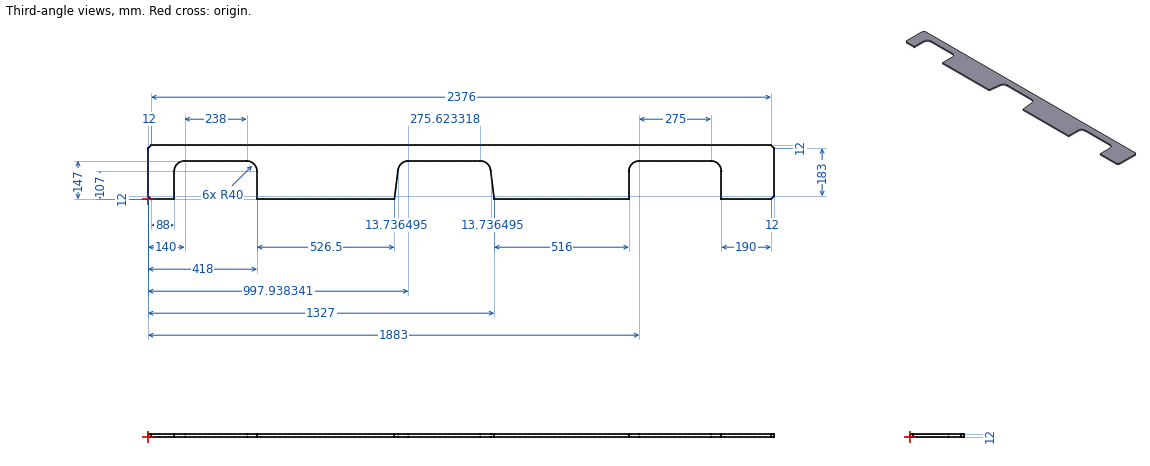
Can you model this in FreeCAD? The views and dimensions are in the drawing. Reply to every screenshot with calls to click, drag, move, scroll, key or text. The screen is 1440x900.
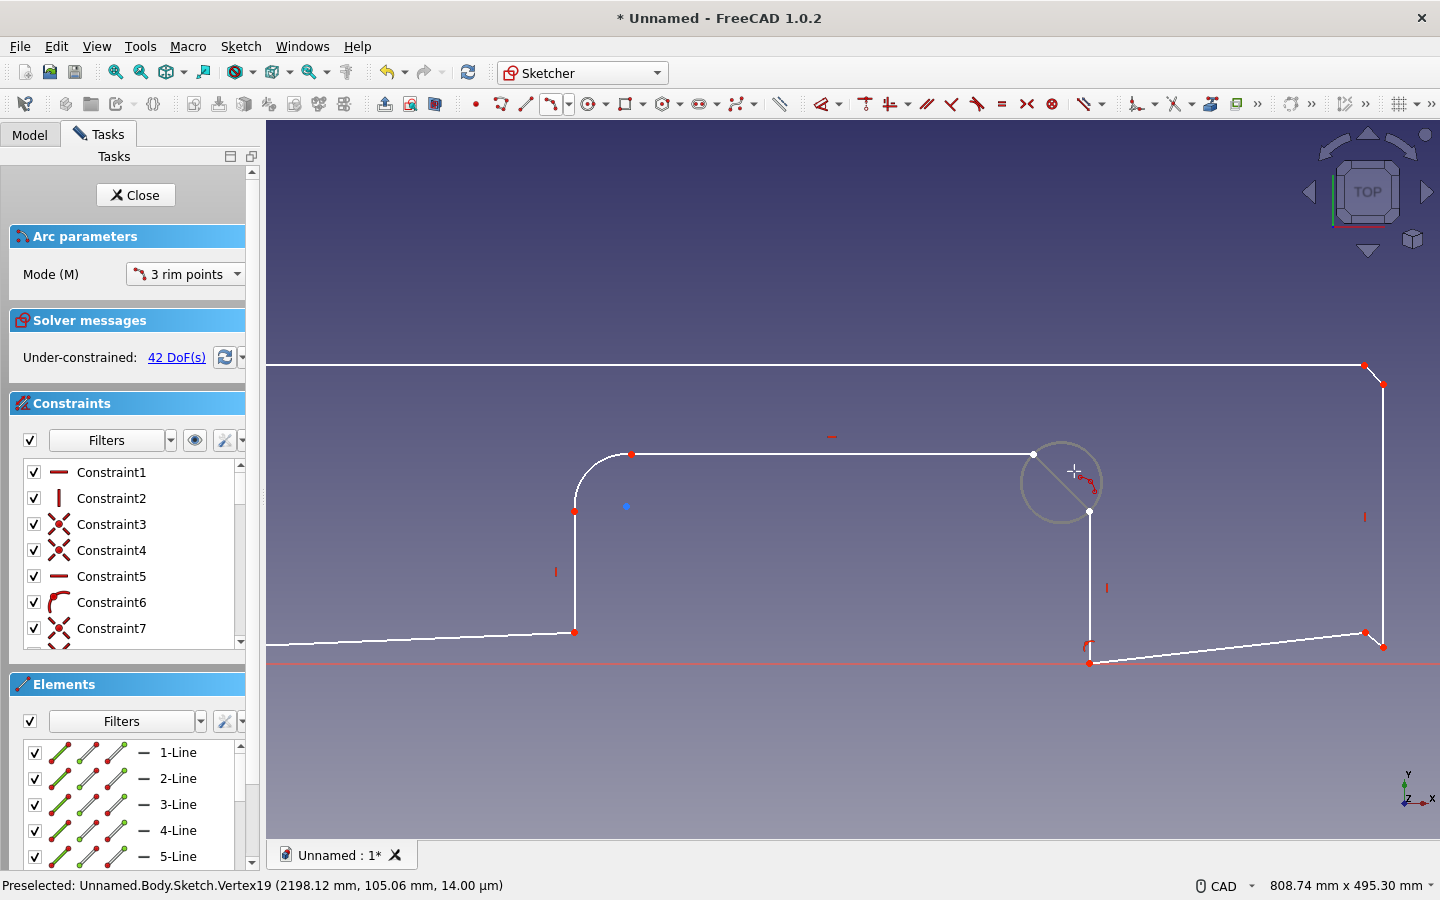
click(1073, 467)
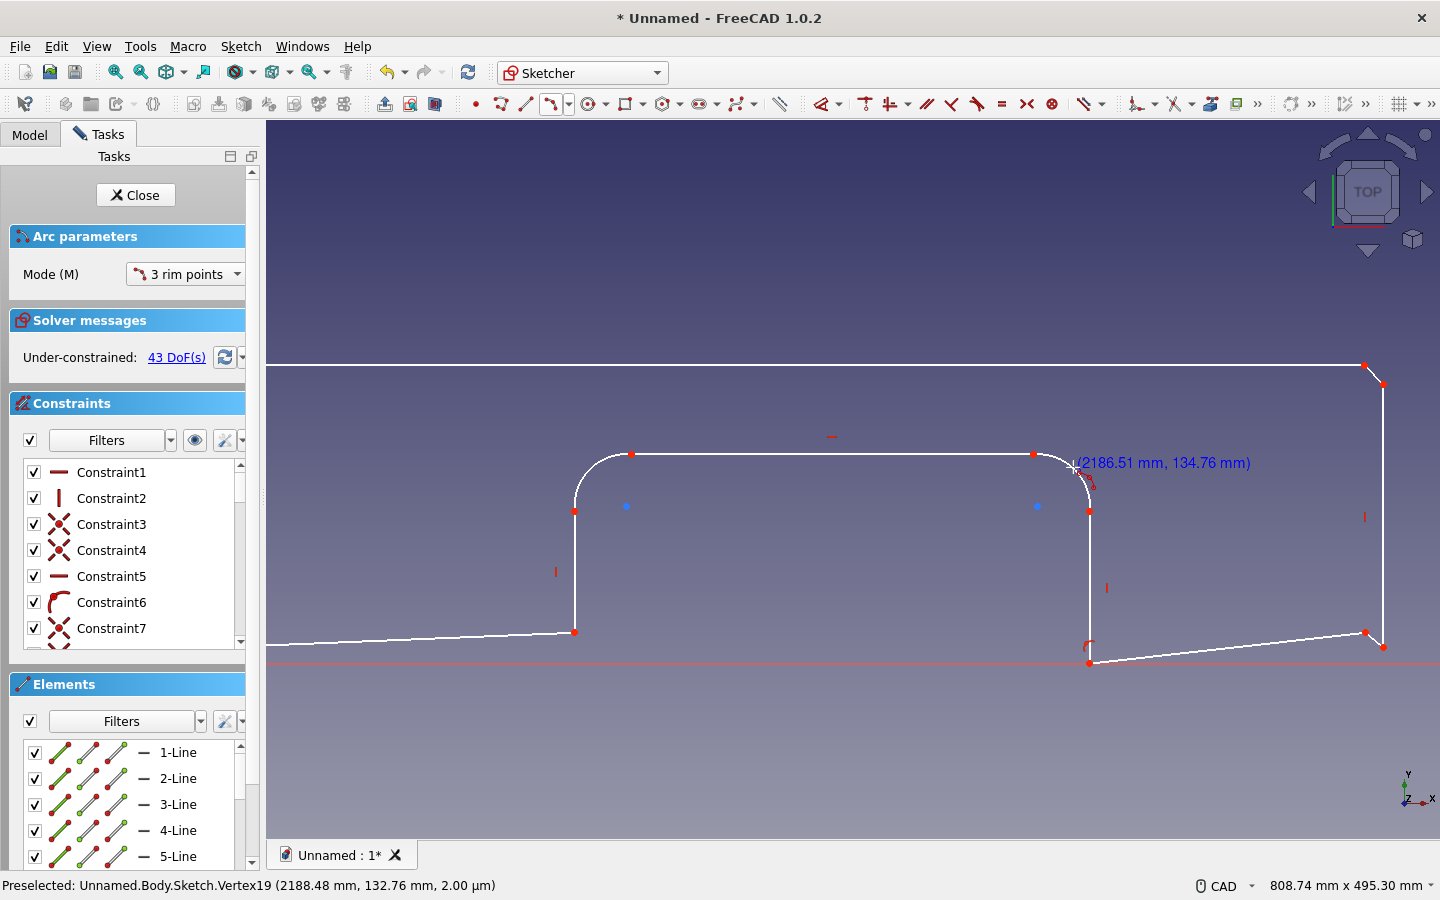
scroll(1074, 471, down, 8)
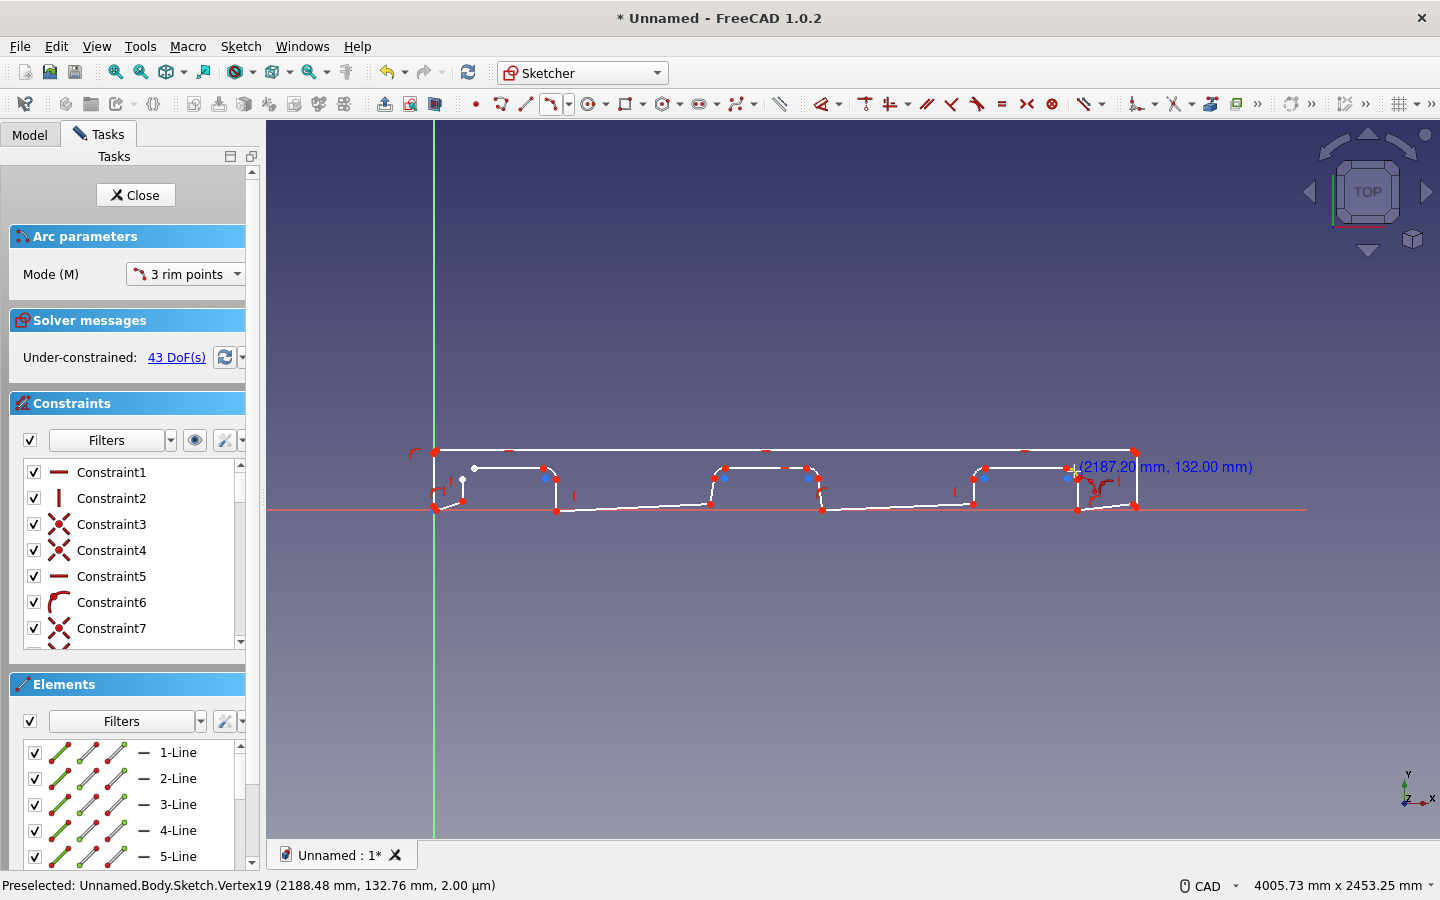
click(463, 480)
click(474, 468)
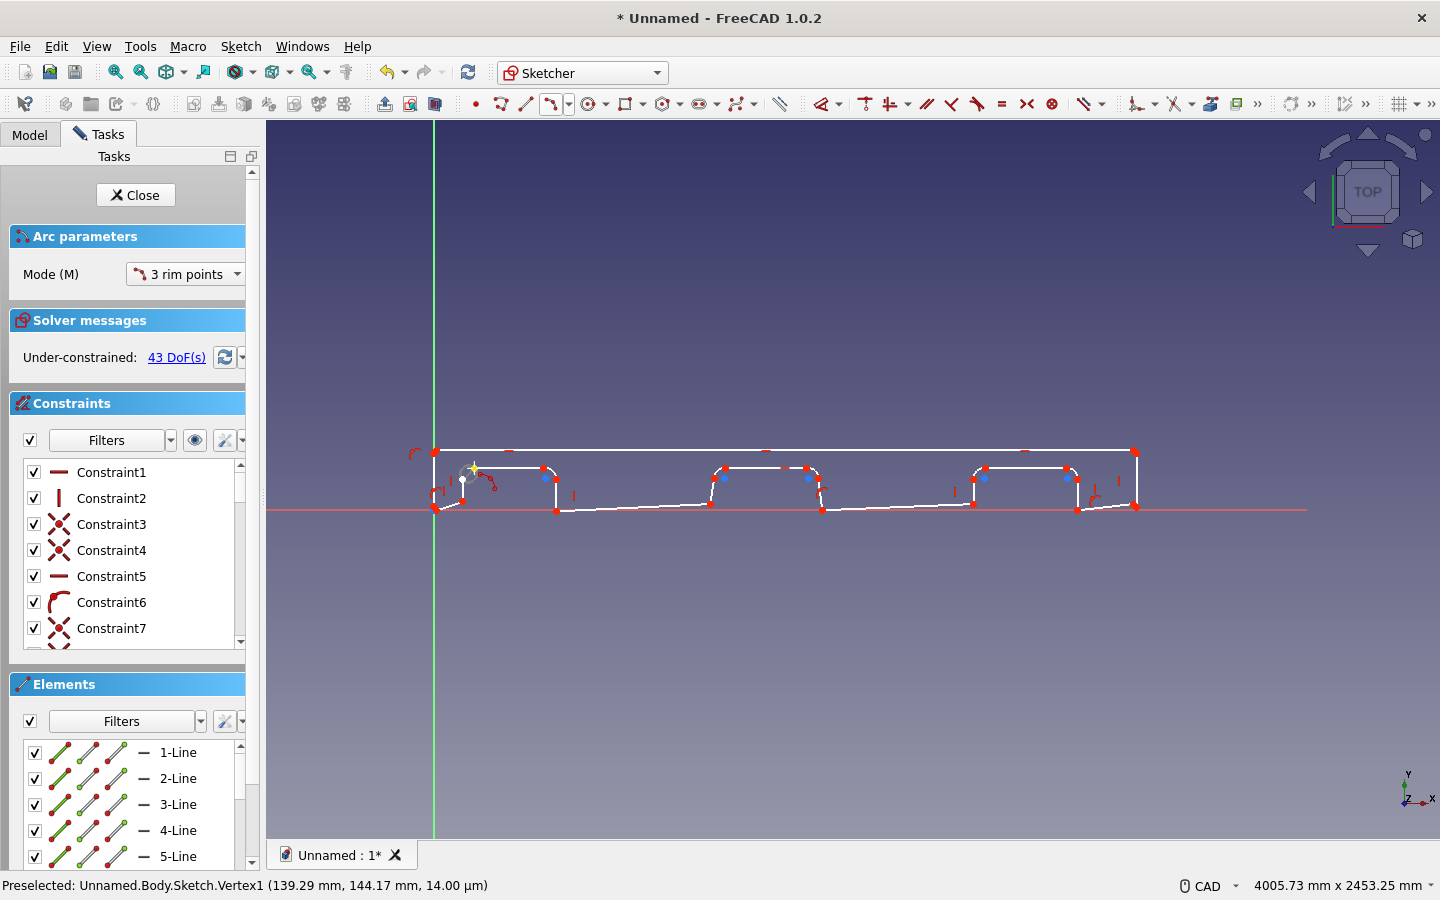
scroll(466, 471, up, 8)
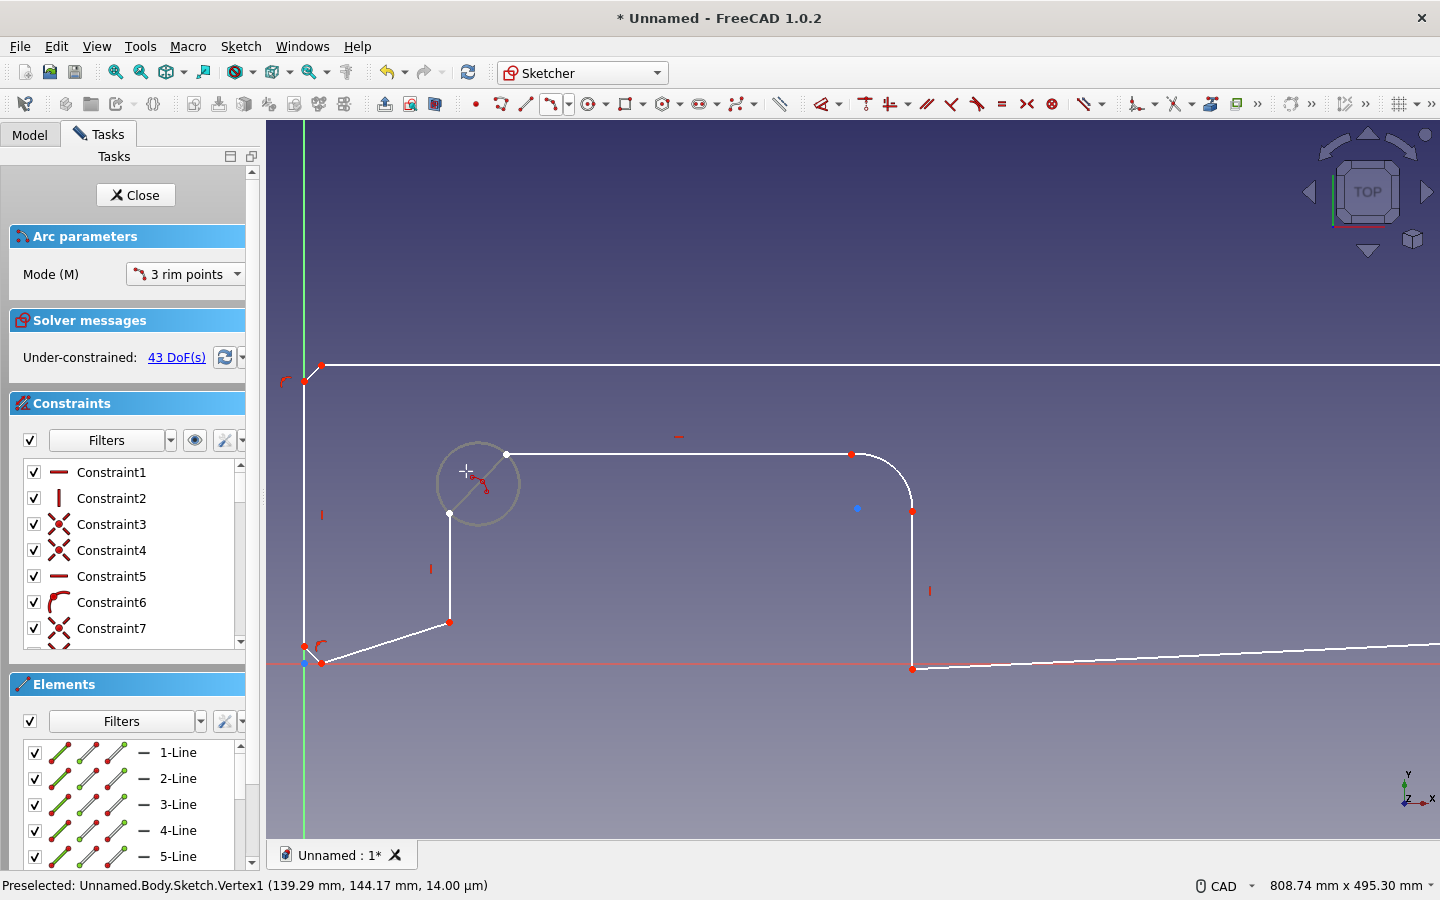
click(467, 467)
key(Escape)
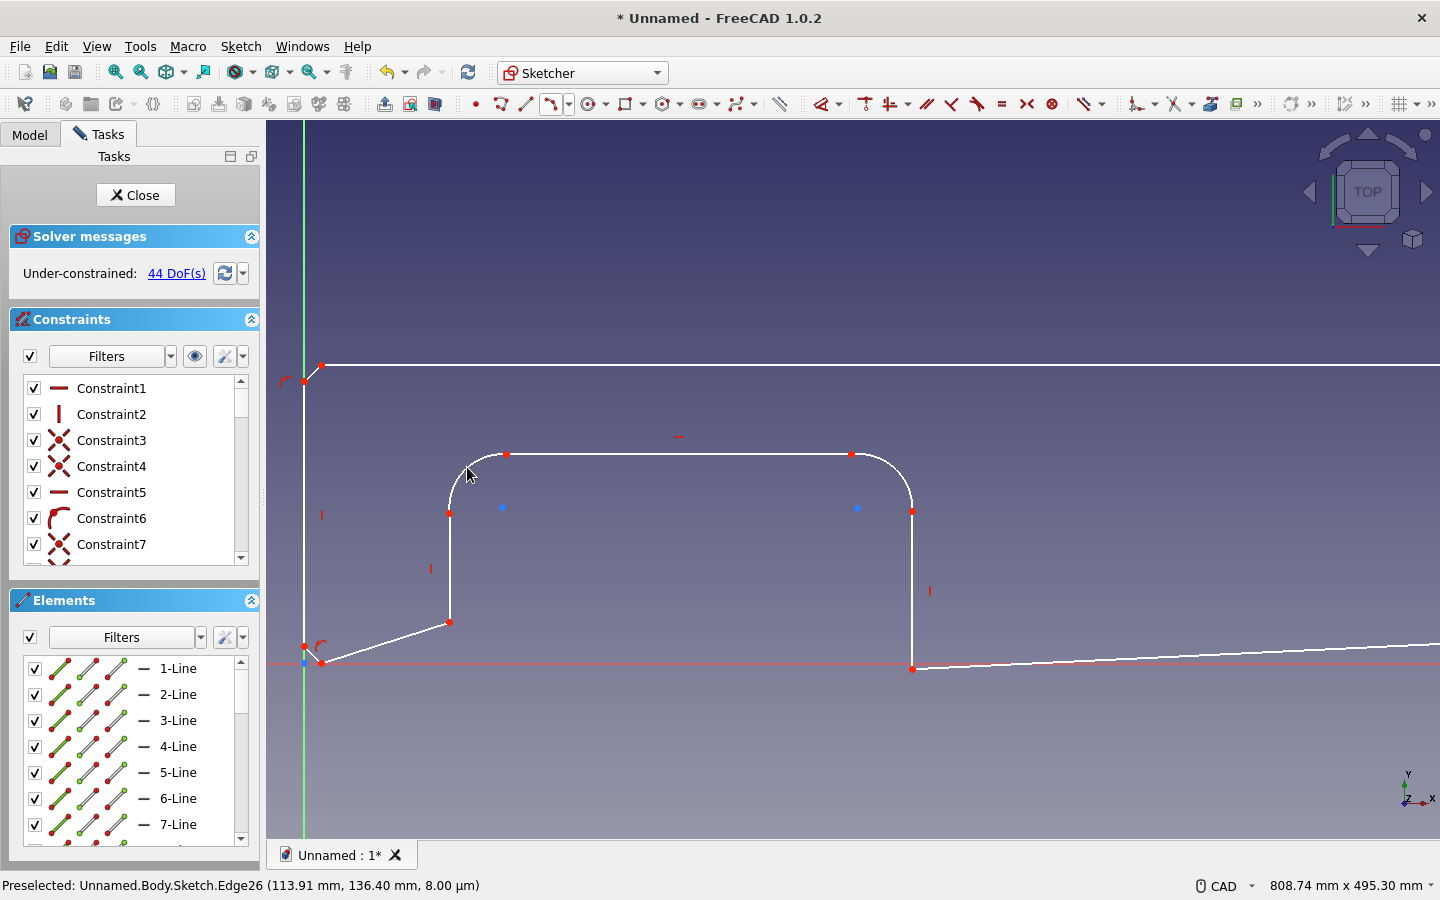
scroll(465, 471, down, 8)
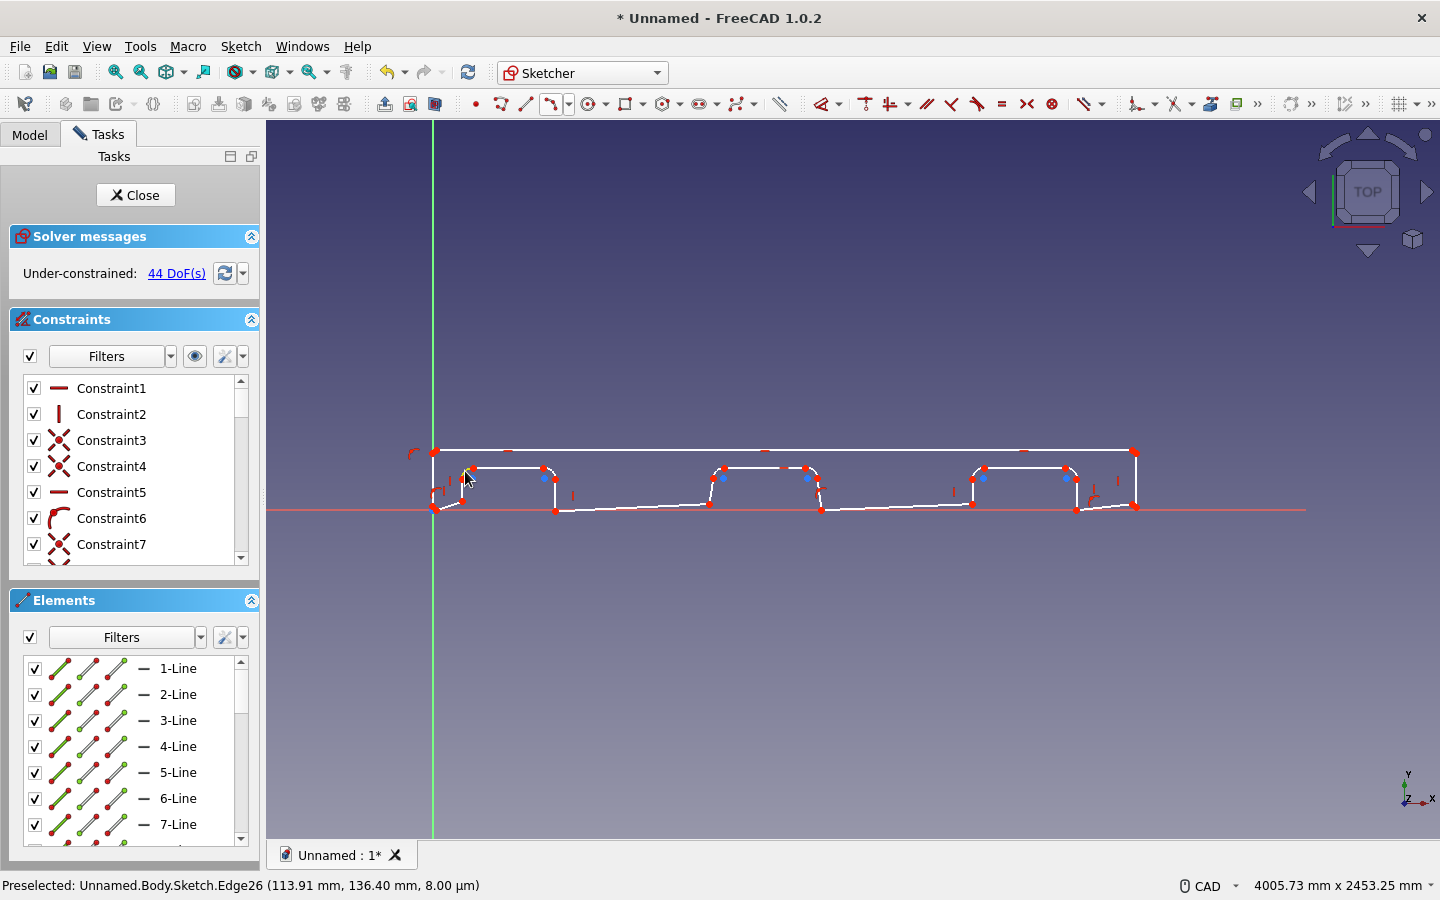
scroll(711, 496, up, 3)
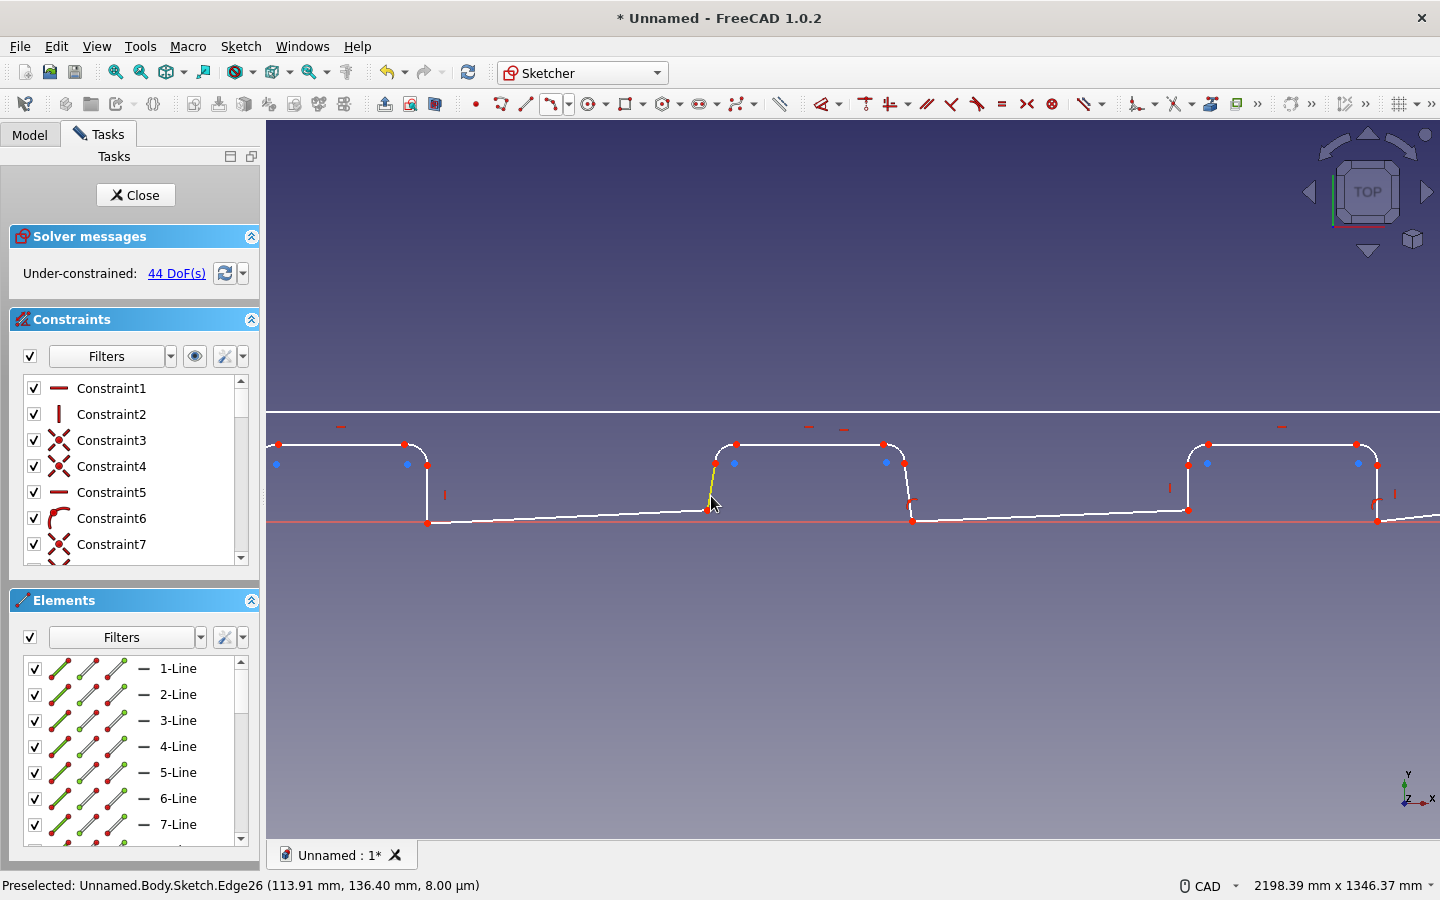
click(710, 496)